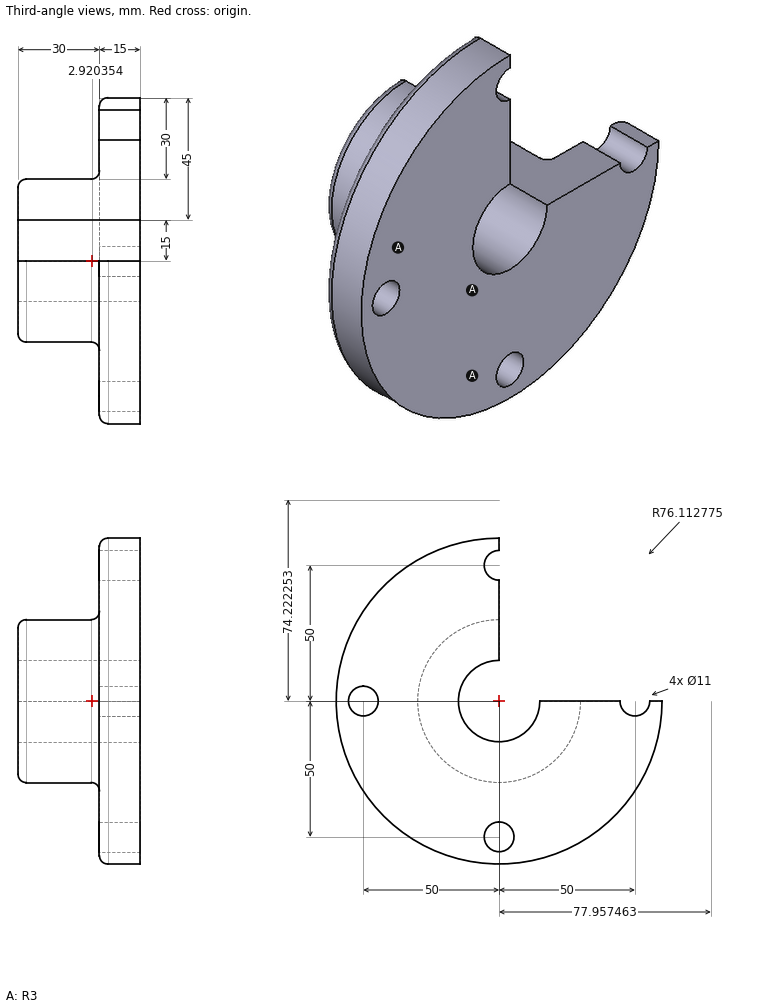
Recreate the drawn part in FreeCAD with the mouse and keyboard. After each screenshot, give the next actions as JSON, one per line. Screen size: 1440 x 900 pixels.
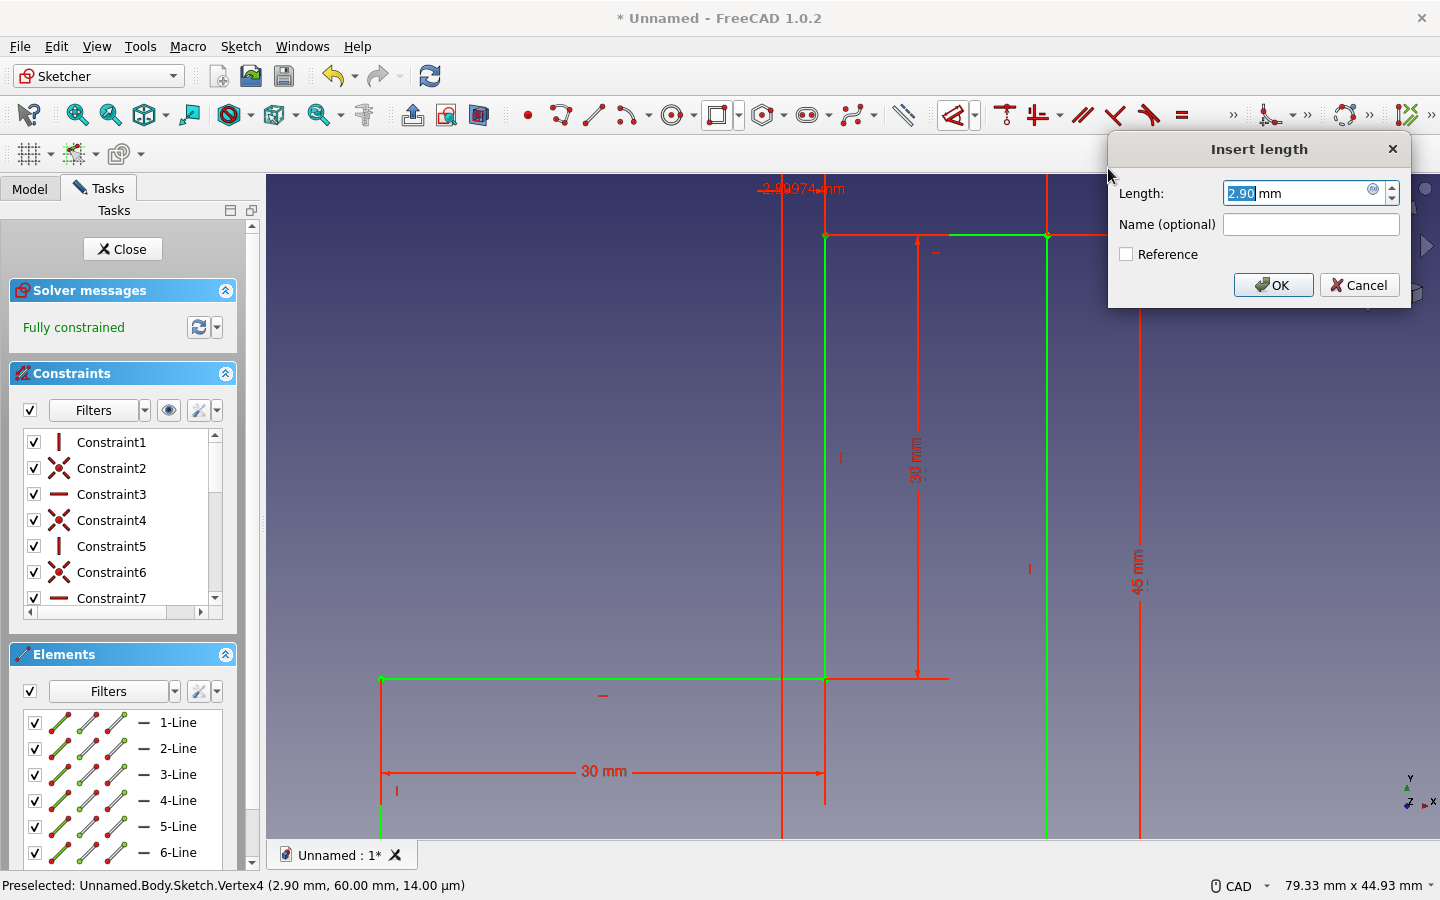
{"action": "type", "text": "2.920354"}
{"action": "key", "text": "Return"}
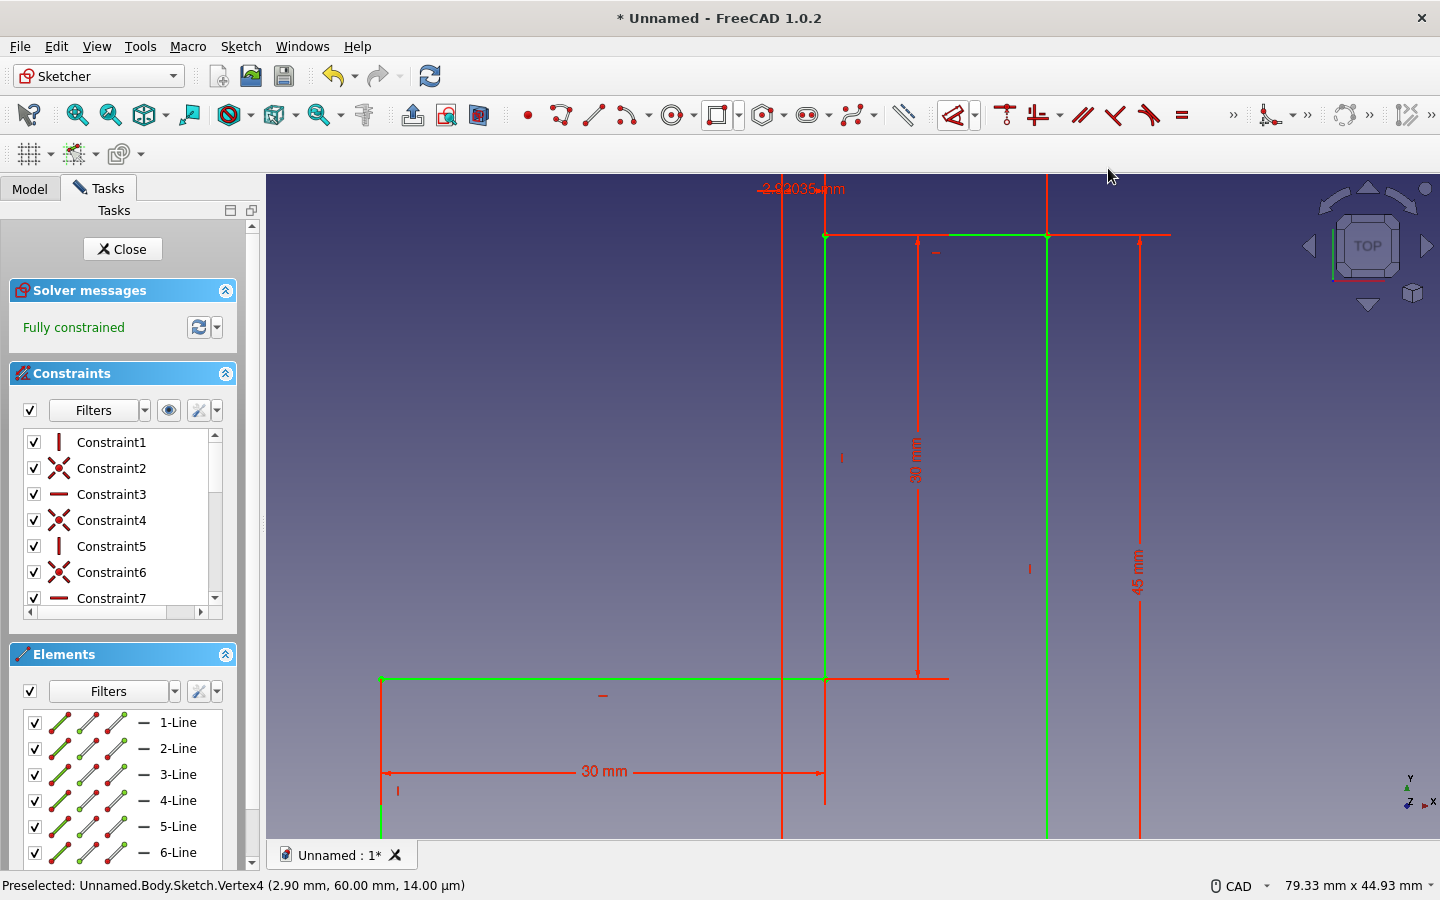
{"action": "left_click", "coordinate": [123, 249]}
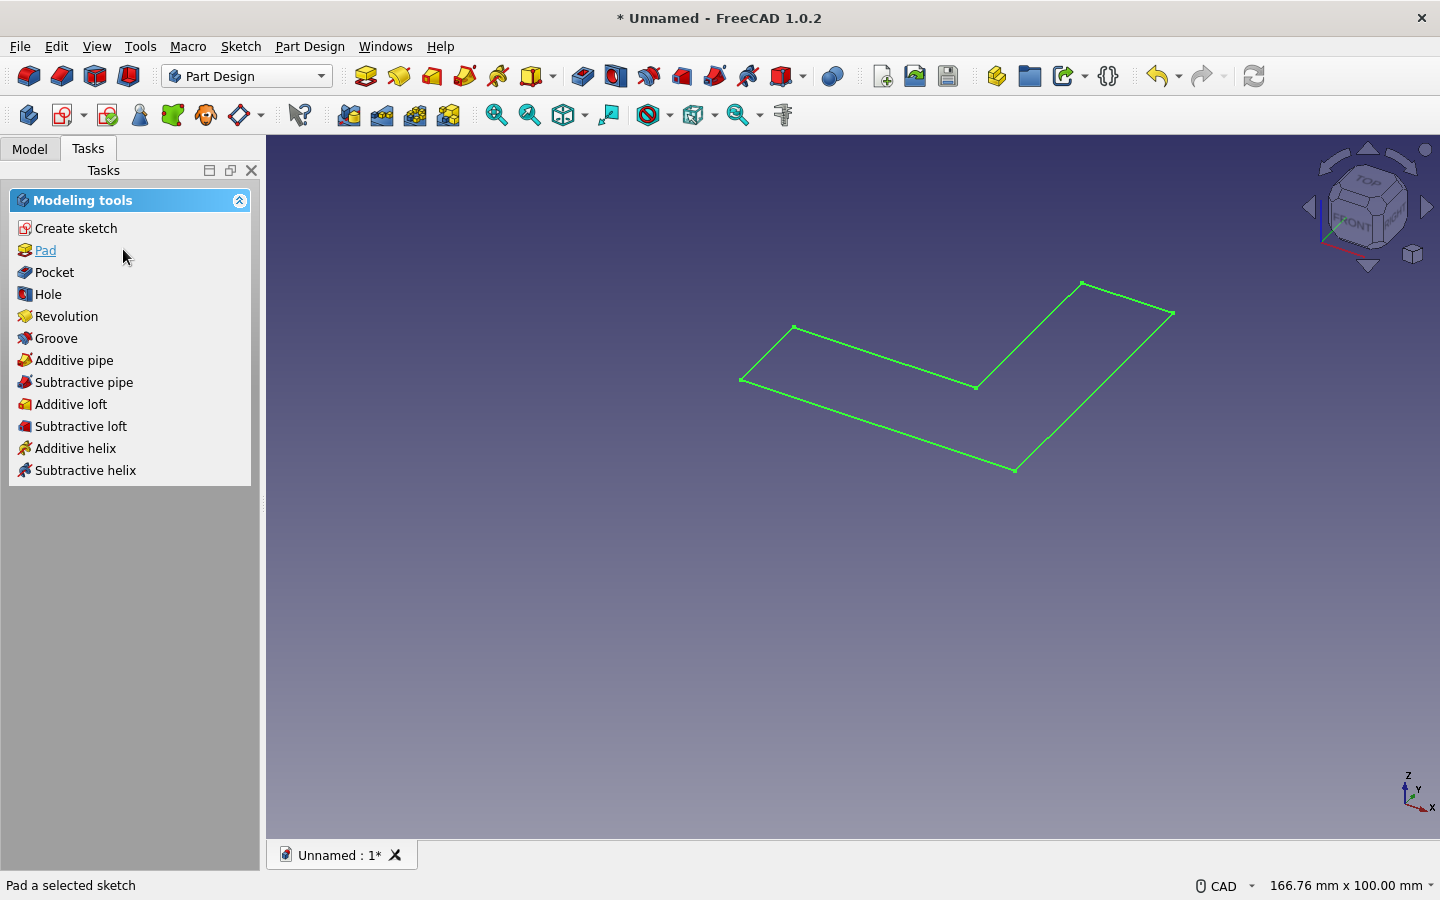
{"action": "left_click", "coordinate": [399, 76]}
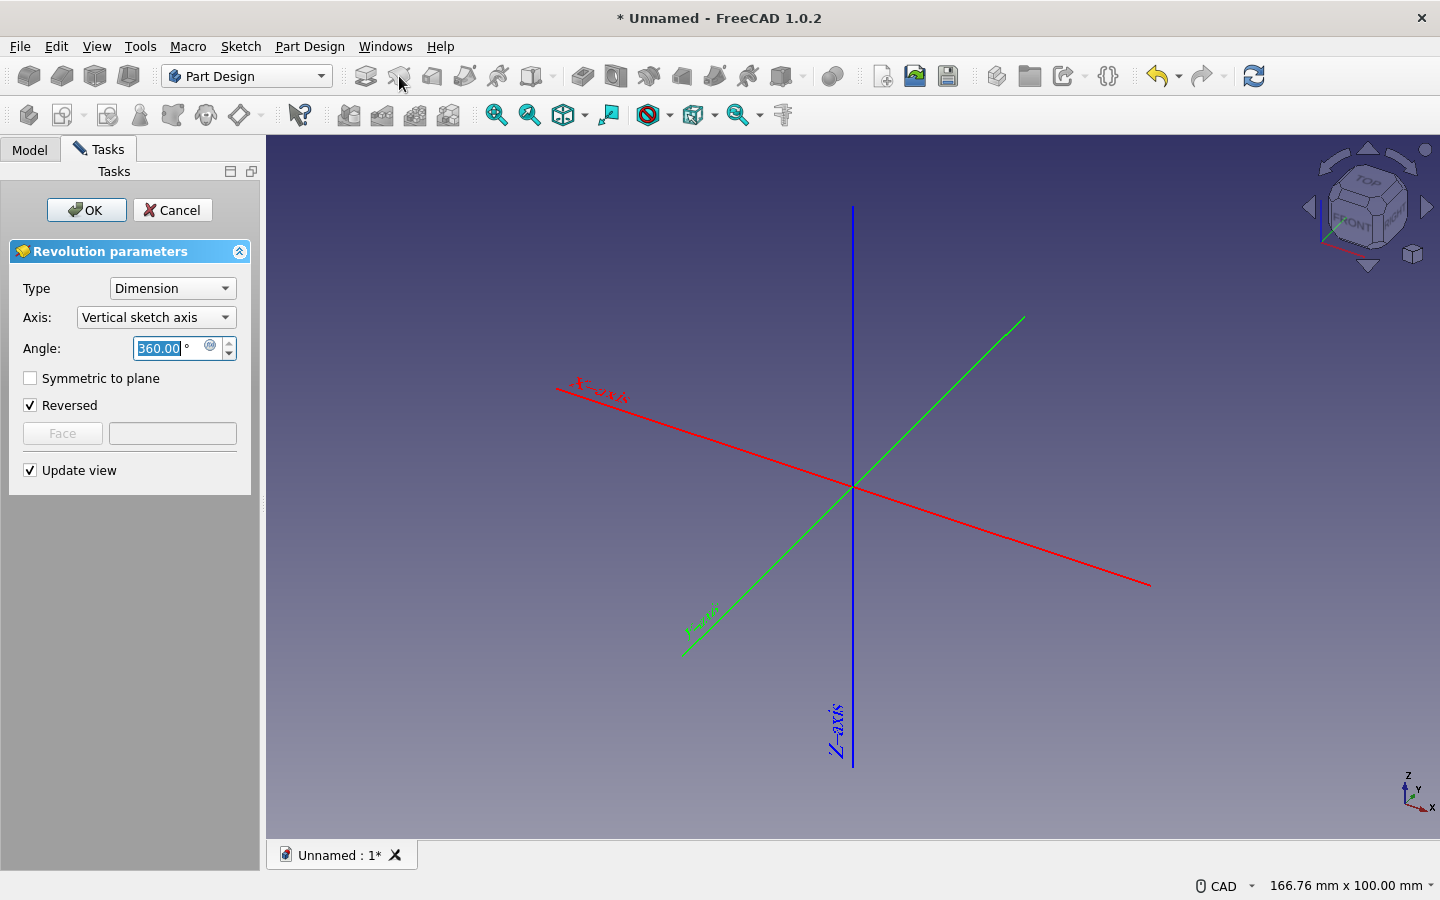
{"action": "left_click", "coordinate": [157, 318]}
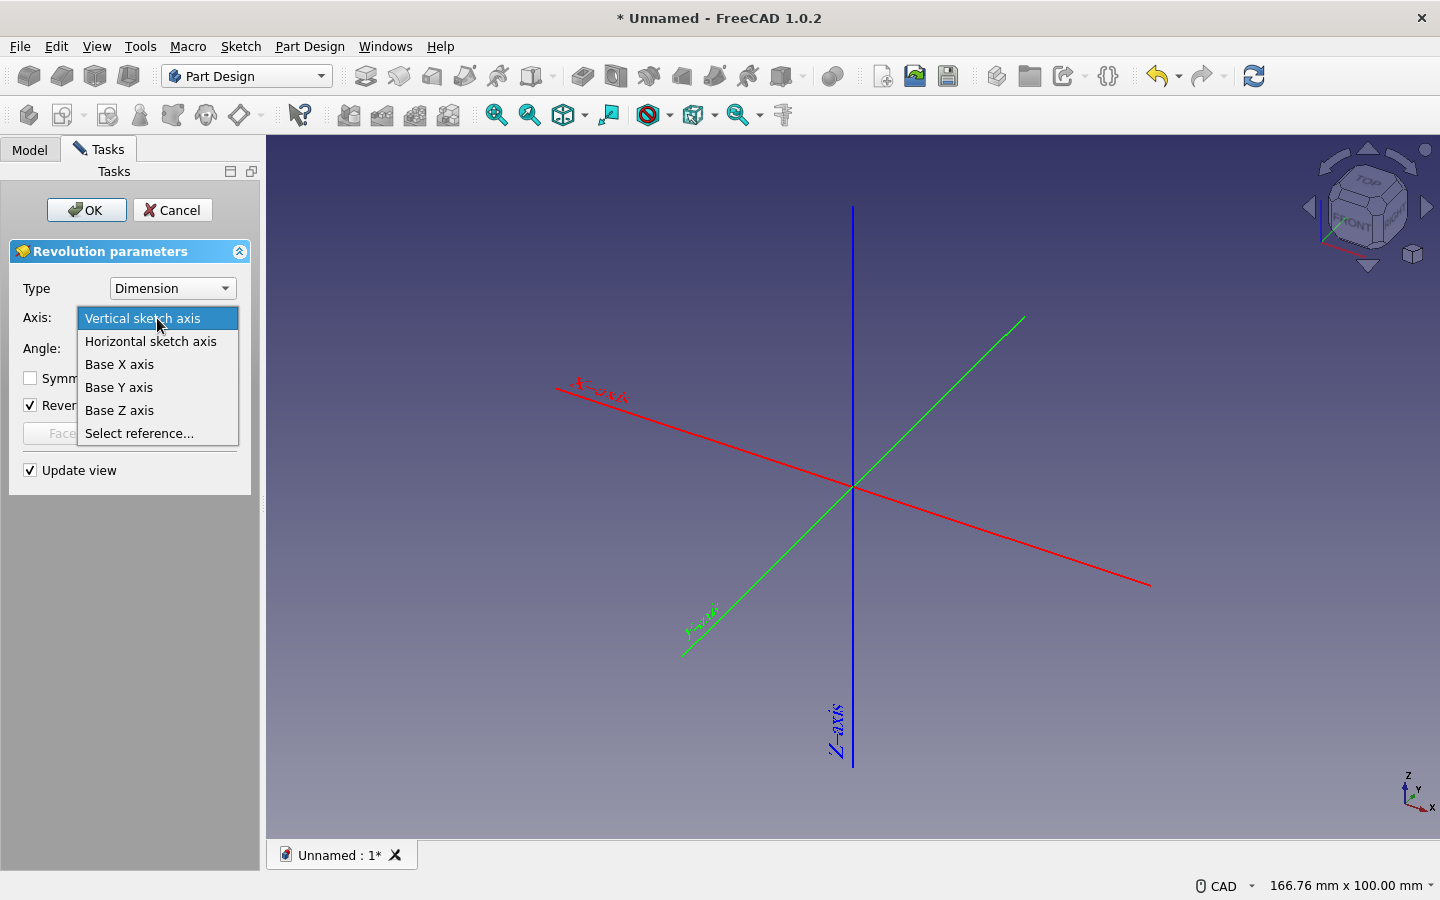
{"action": "left_click", "coordinate": [156, 342]}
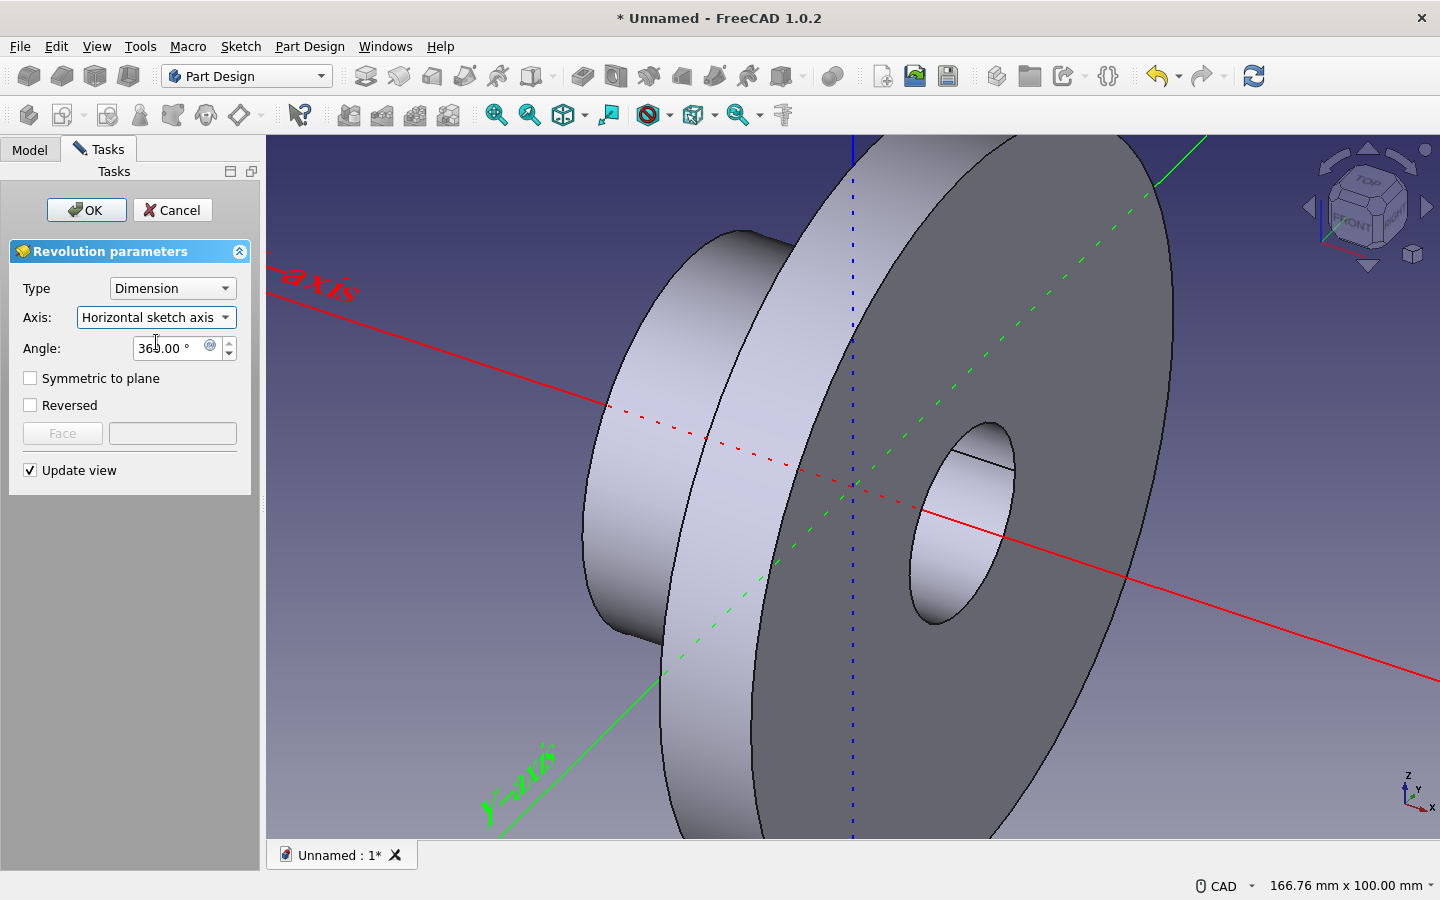
{"action": "left_click", "coordinate": [87, 210]}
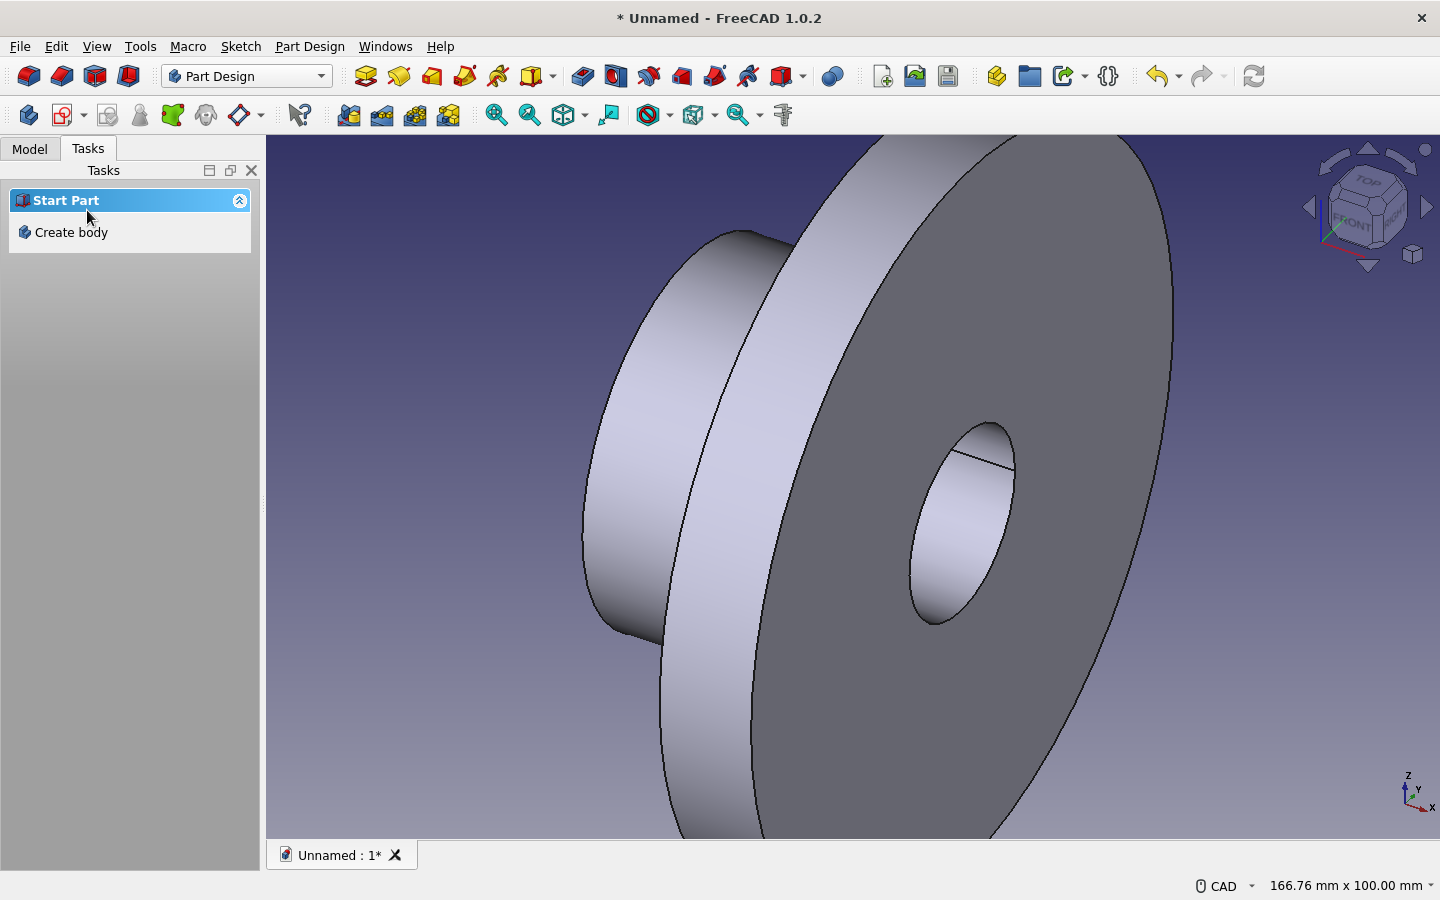
{"action": "left_click", "coordinate": [497, 116]}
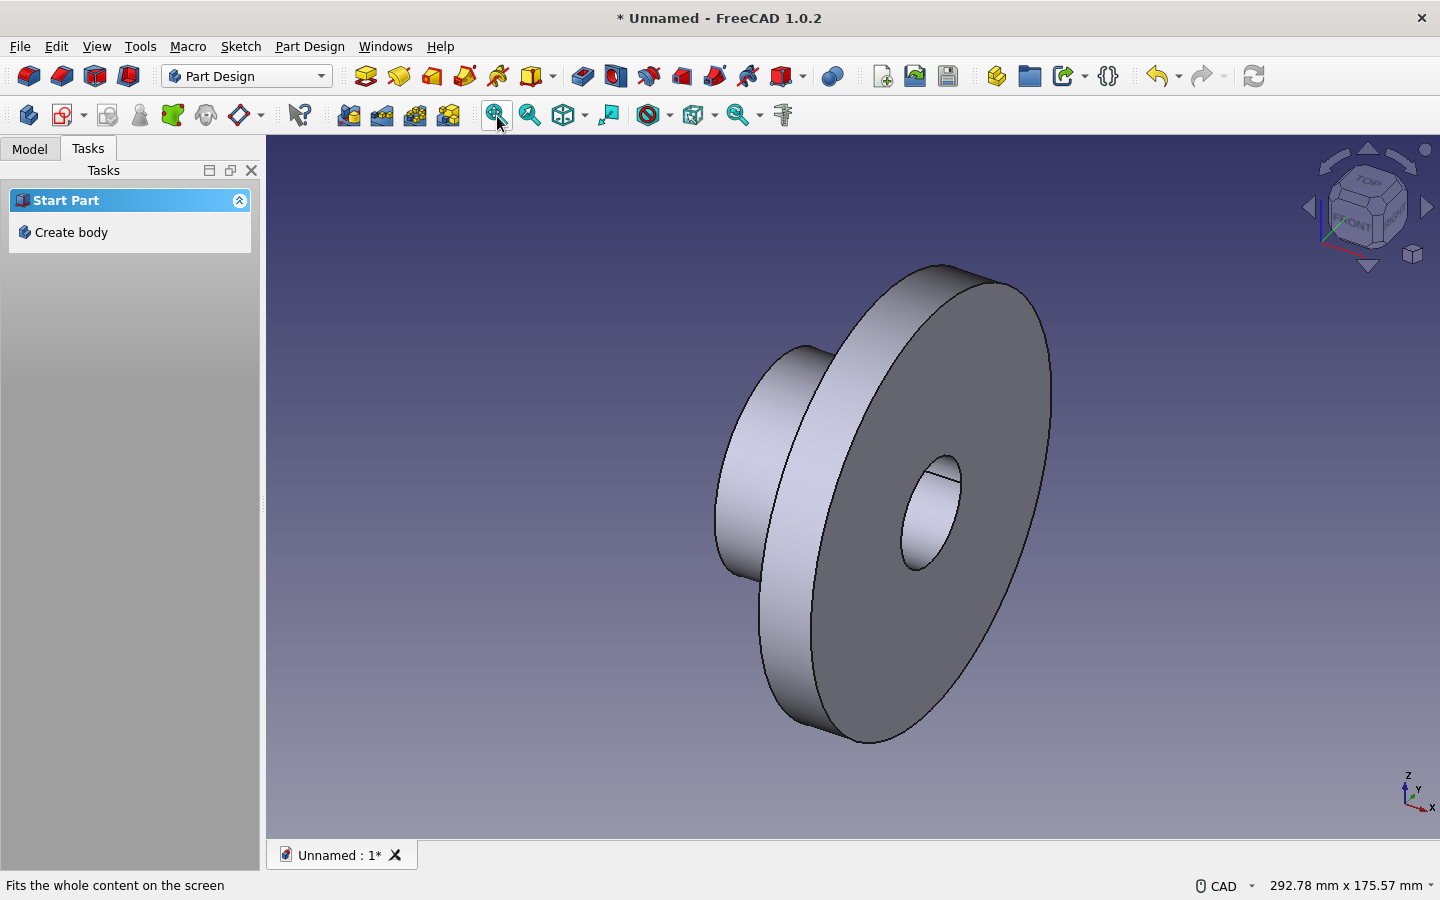
{"action": "key", "text": "6"}